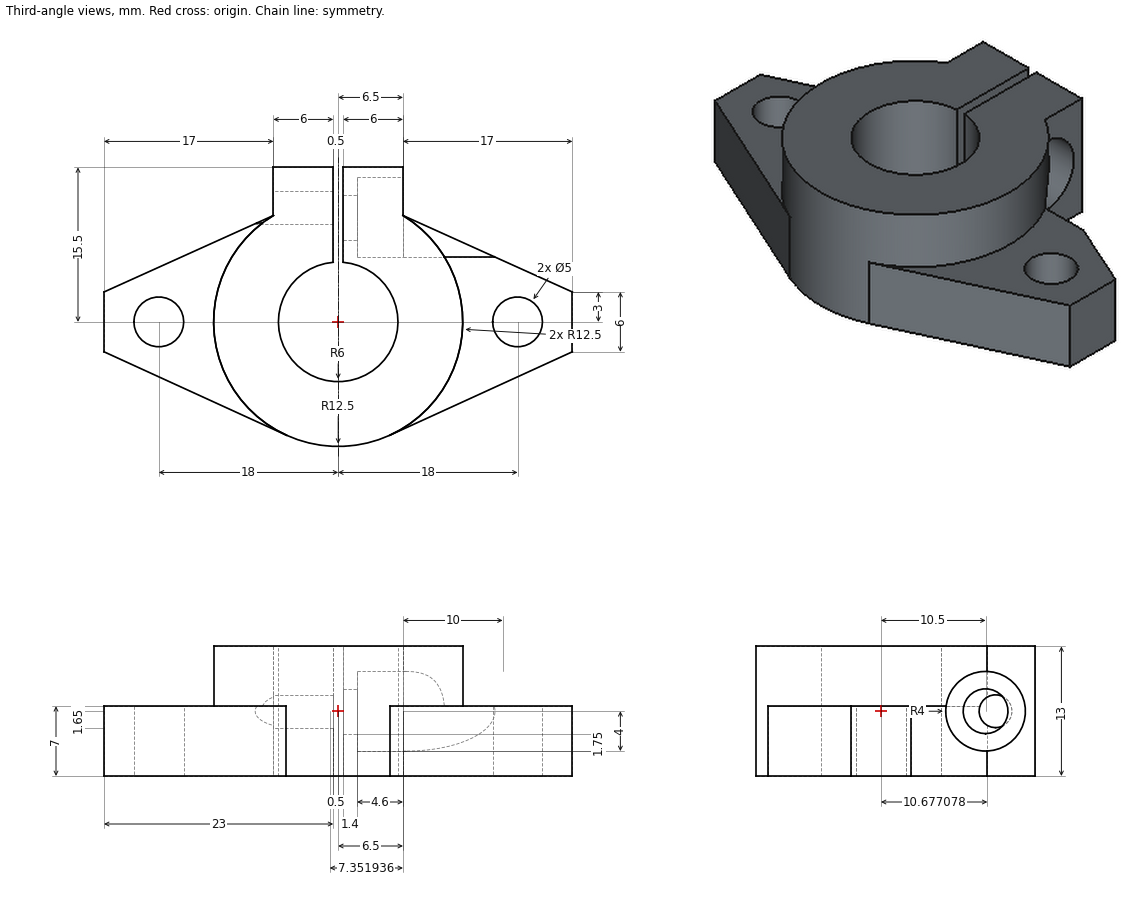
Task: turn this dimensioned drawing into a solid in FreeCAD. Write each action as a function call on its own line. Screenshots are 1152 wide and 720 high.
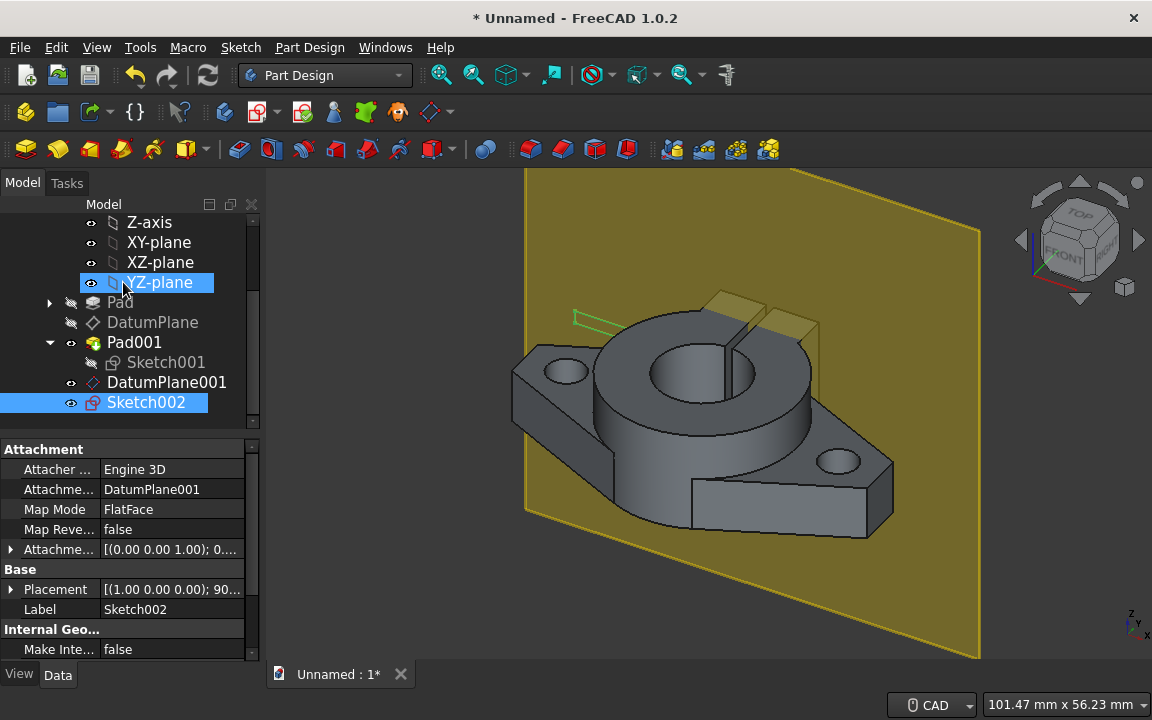
click(304, 150)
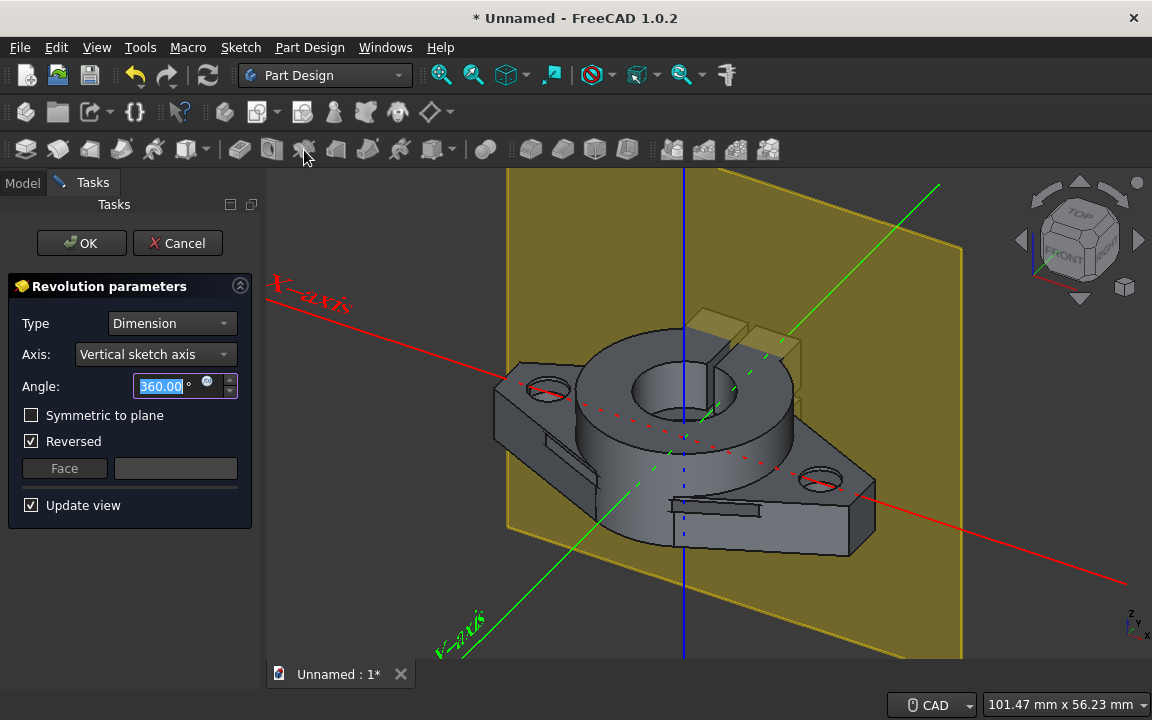
click(156, 354)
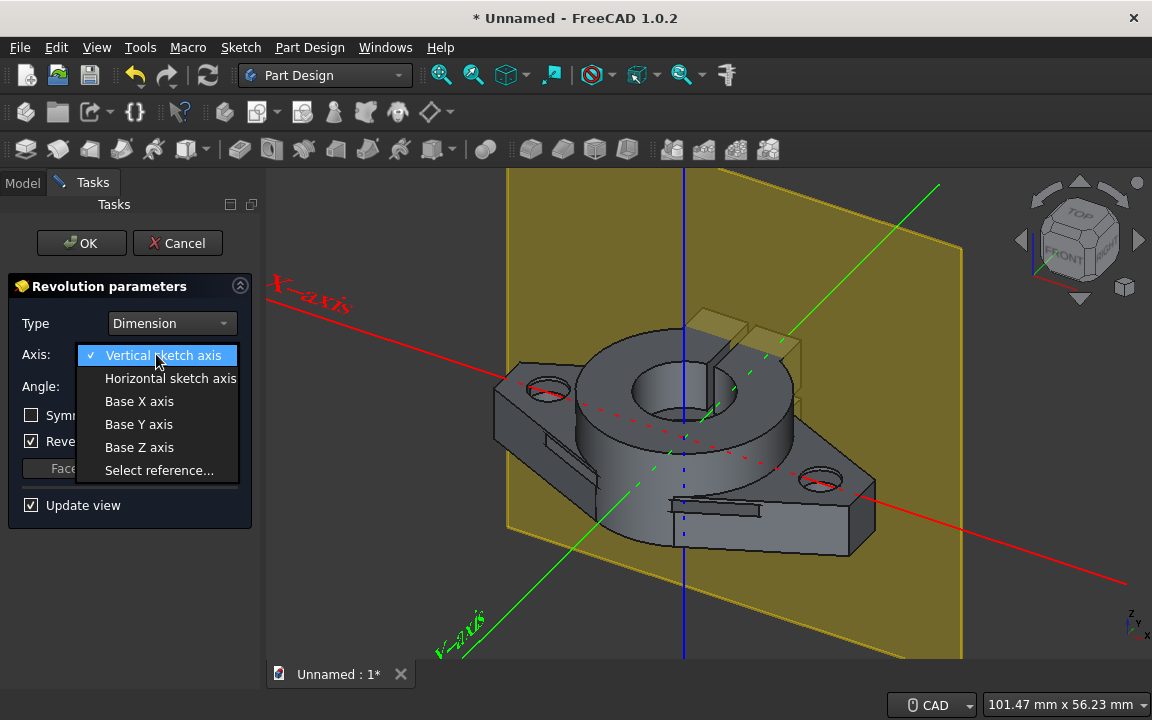
click(156, 378)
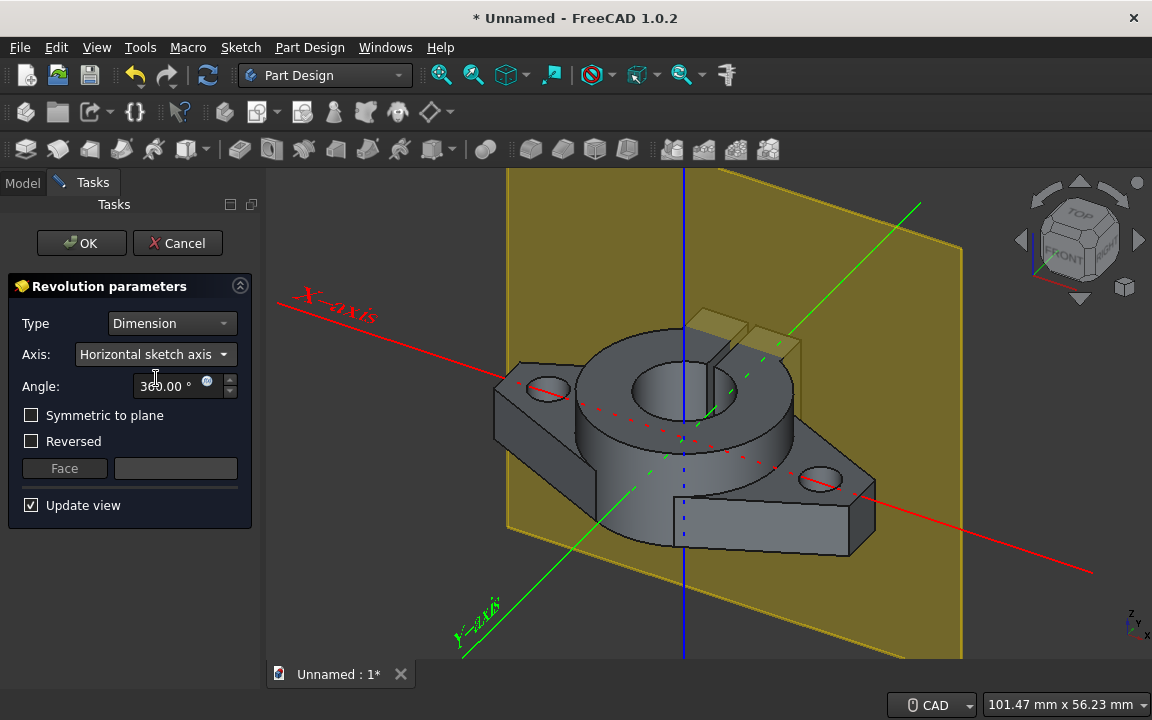
click(82, 243)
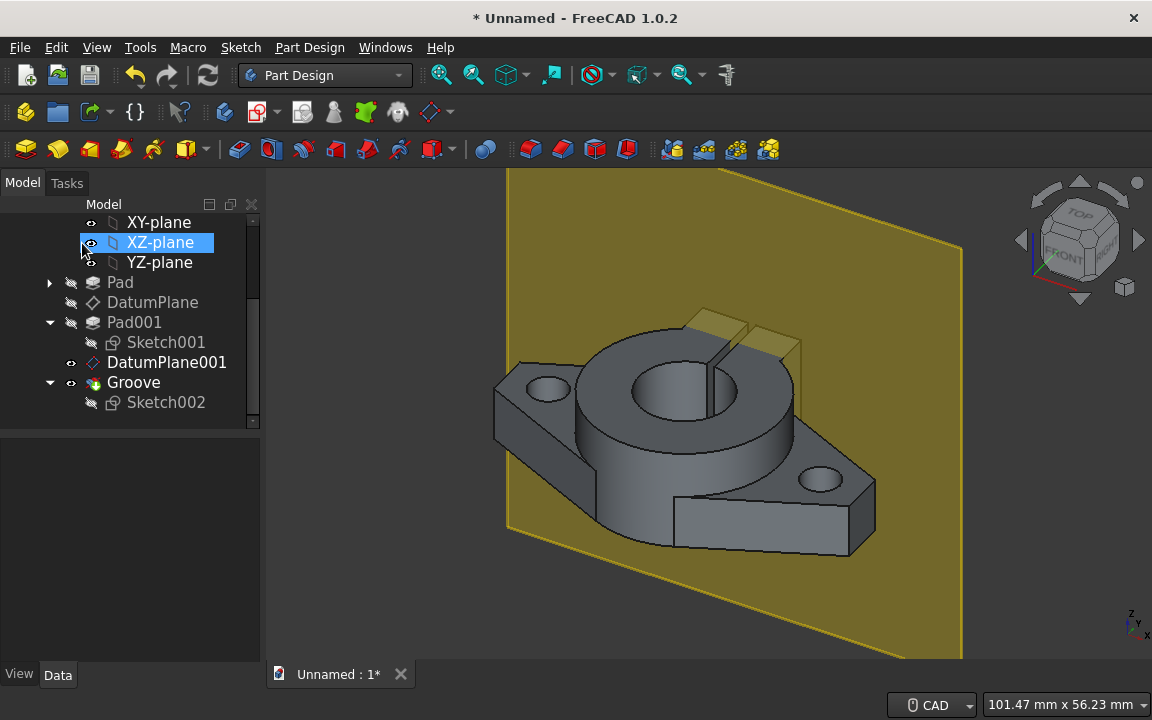
click(116, 363)
key(space)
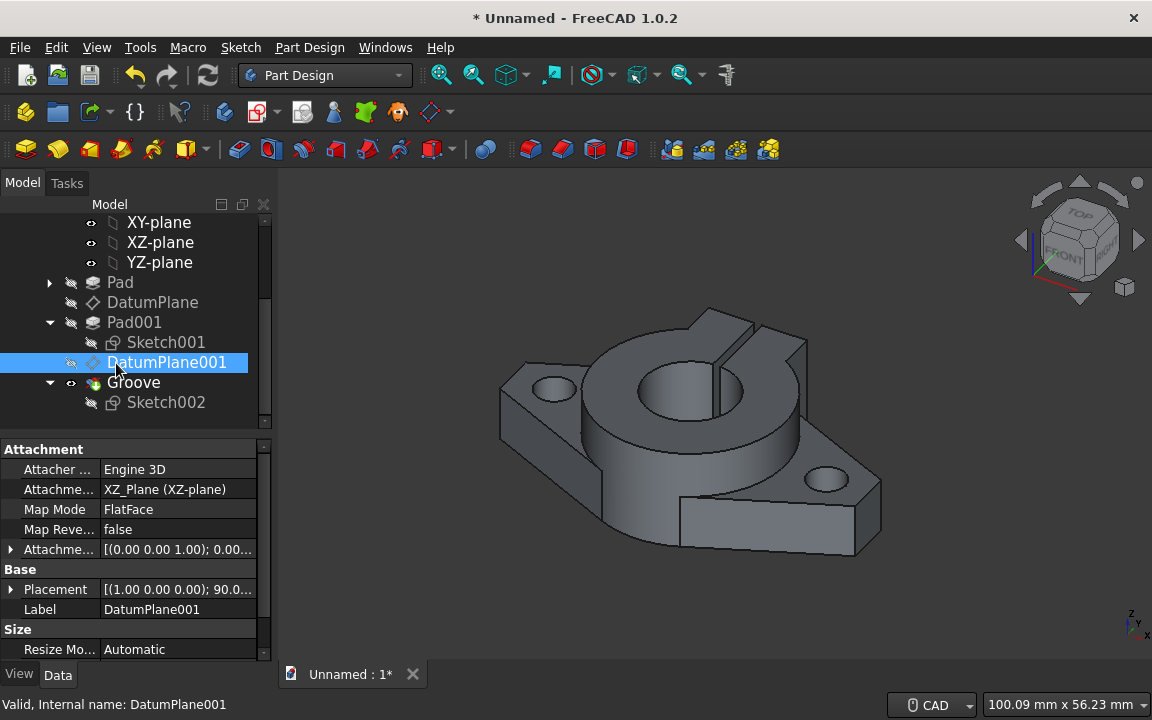
scroll(160, 318, down, 3)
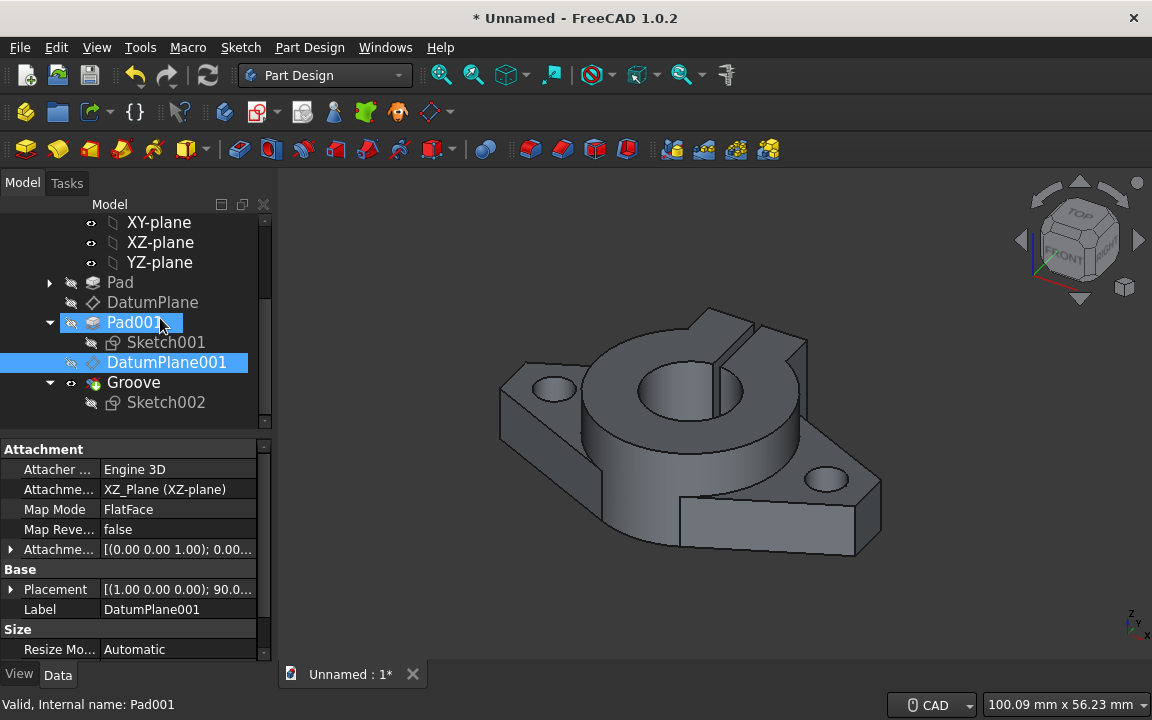
scroll(160, 318, up, 15)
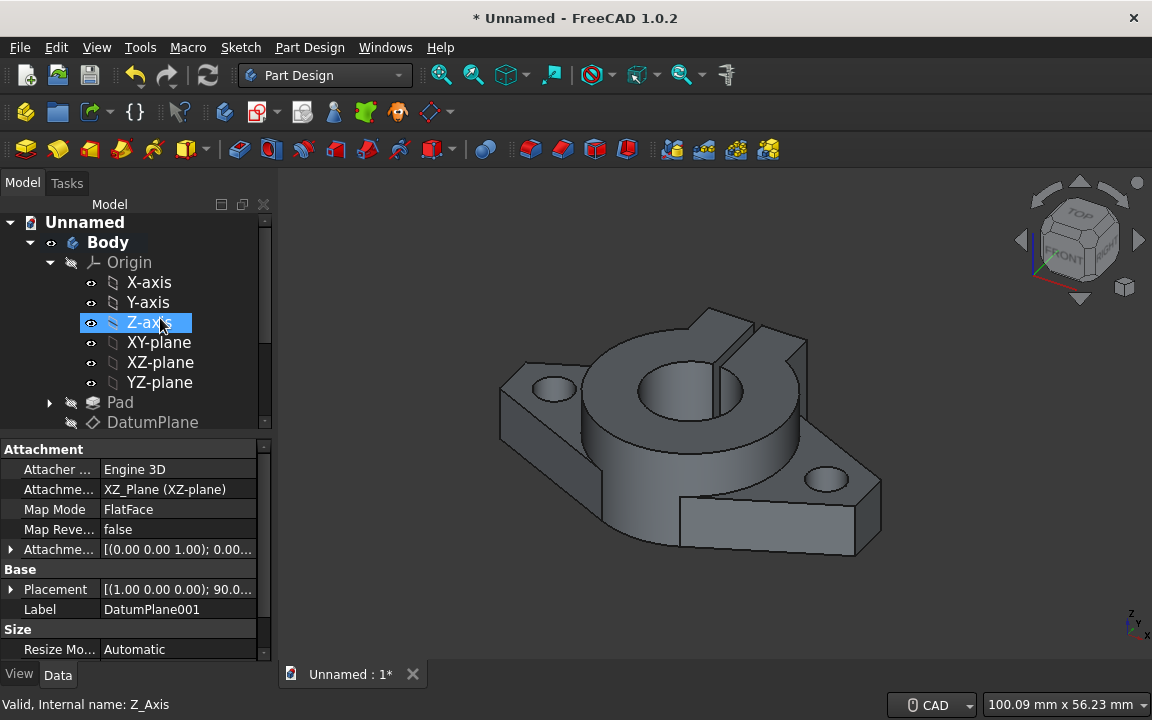
click(136, 363)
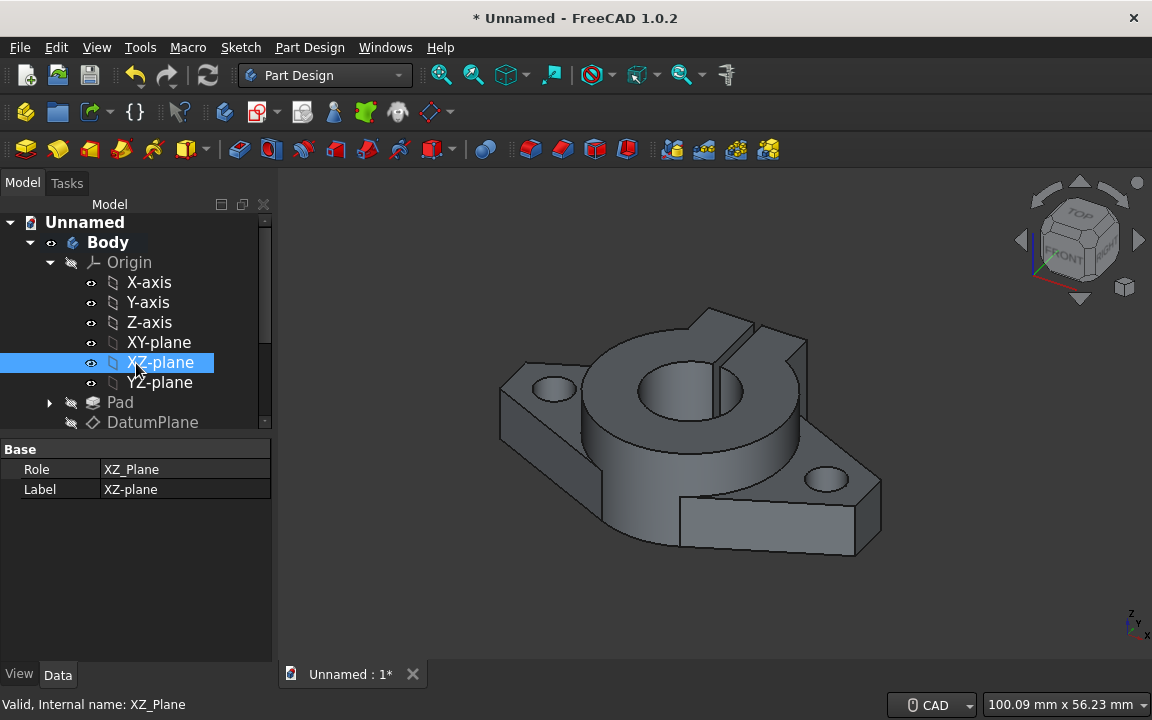
click(430, 112)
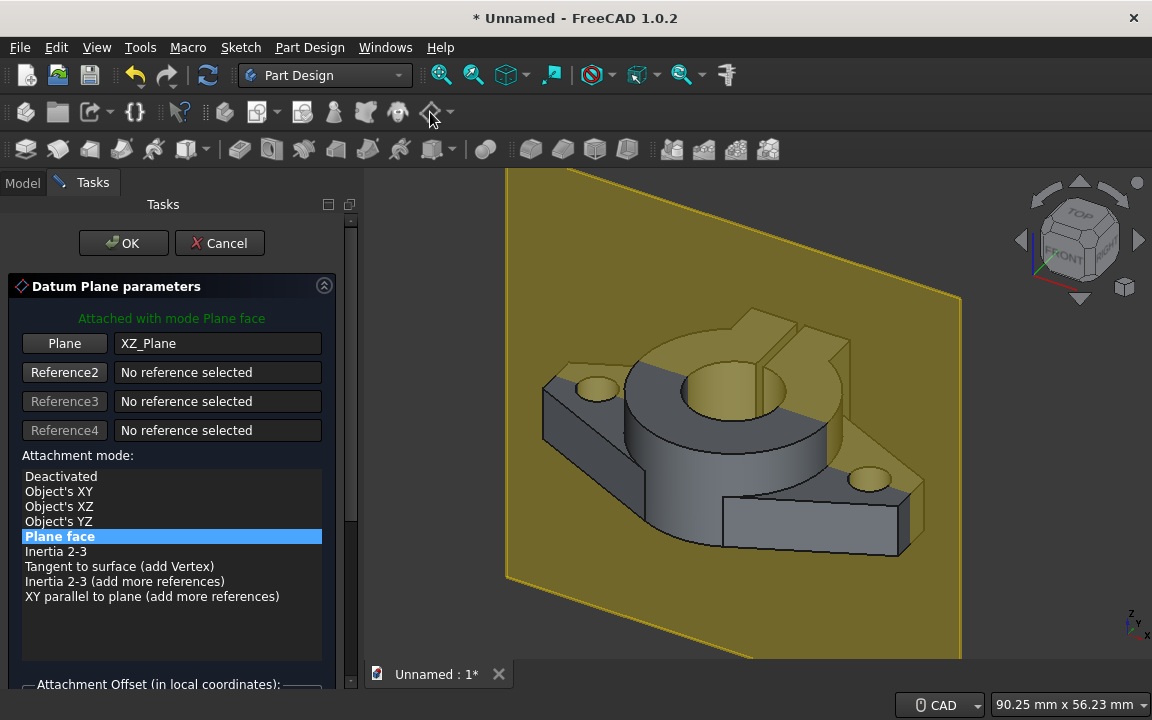
scroll(351, 451, down, 3)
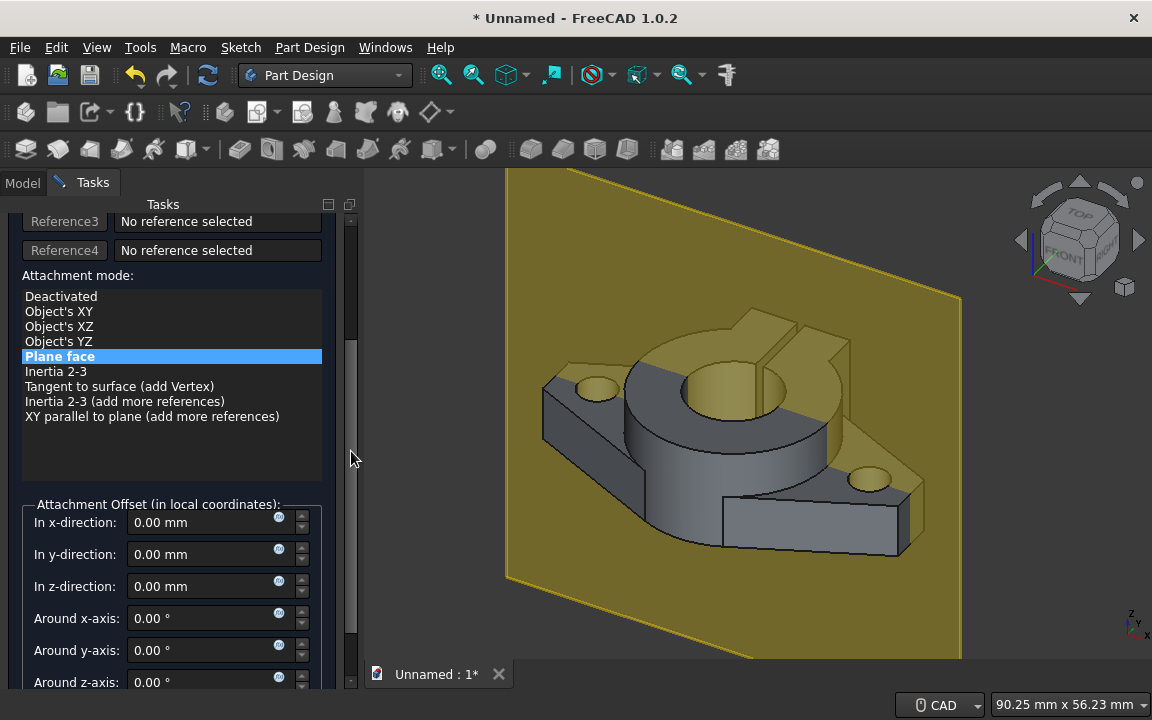
triple_click(210, 586)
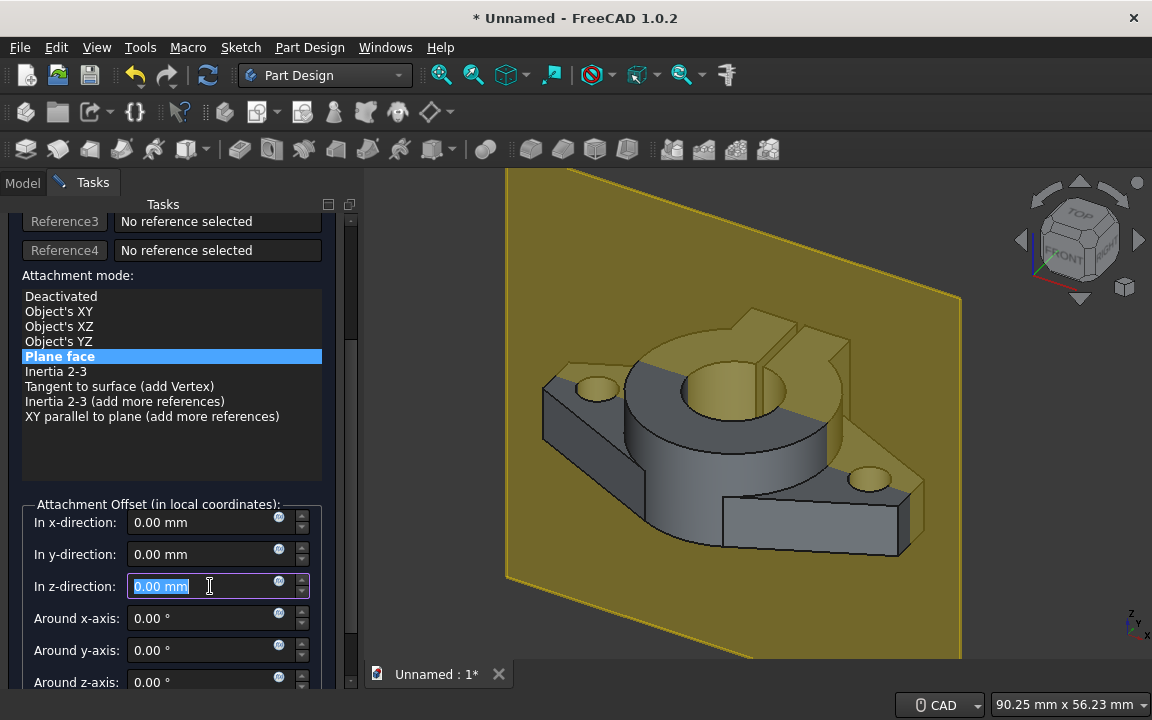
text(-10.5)
key(Tab)